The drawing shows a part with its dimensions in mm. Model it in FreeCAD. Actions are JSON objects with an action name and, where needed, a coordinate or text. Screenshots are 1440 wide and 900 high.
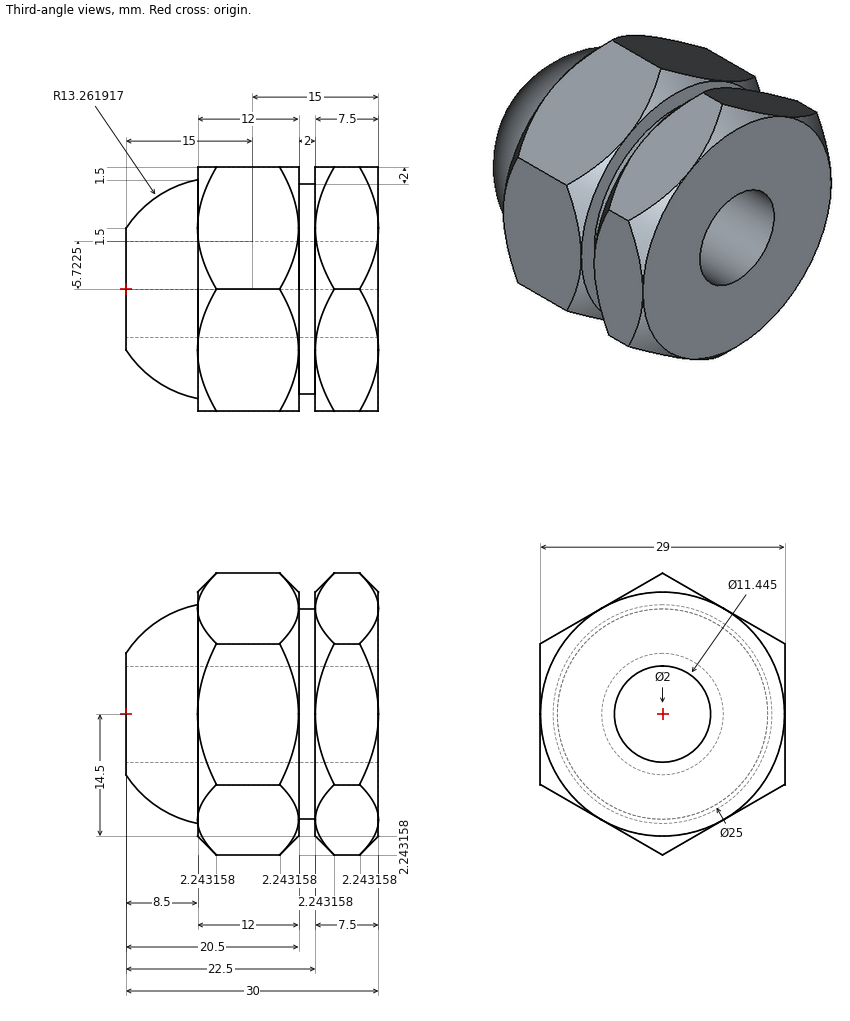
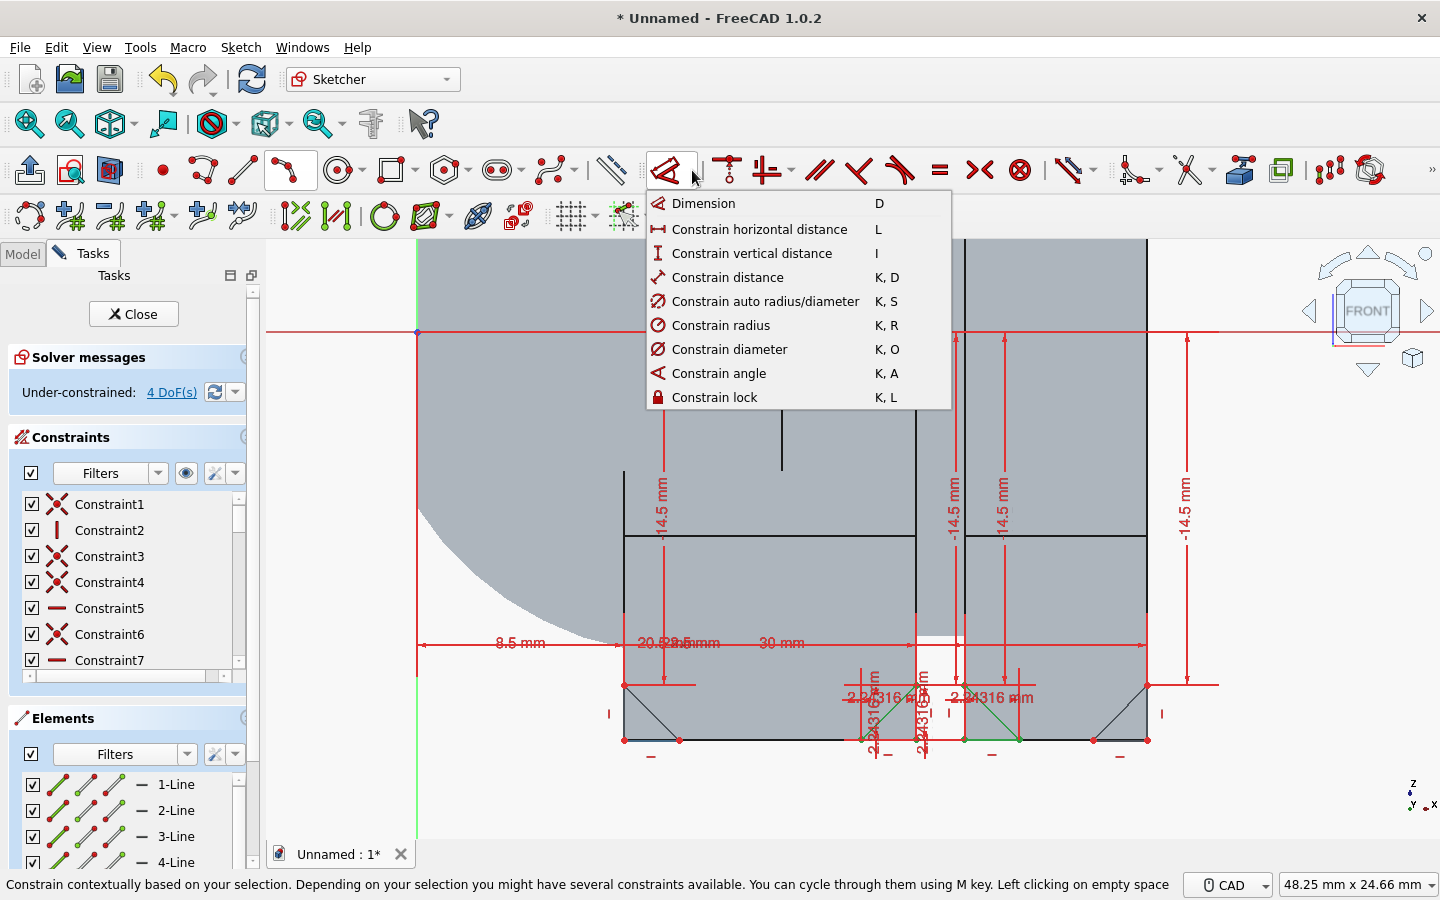
{"action": "left_click", "coordinate": [799, 229]}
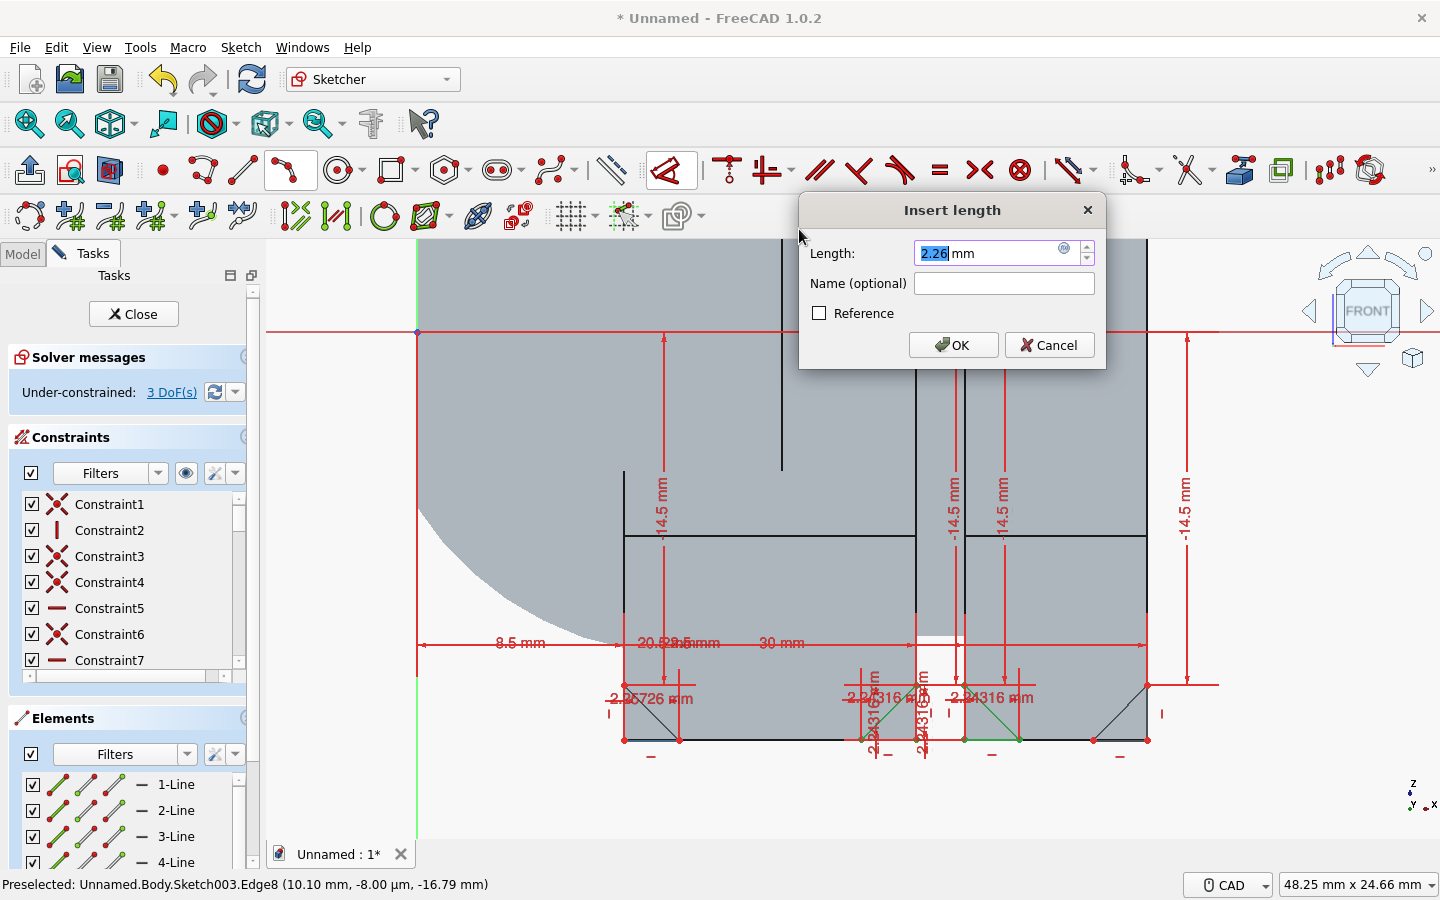
{"action": "type", "text": "2.243158"}
{"action": "key", "text": "Return"}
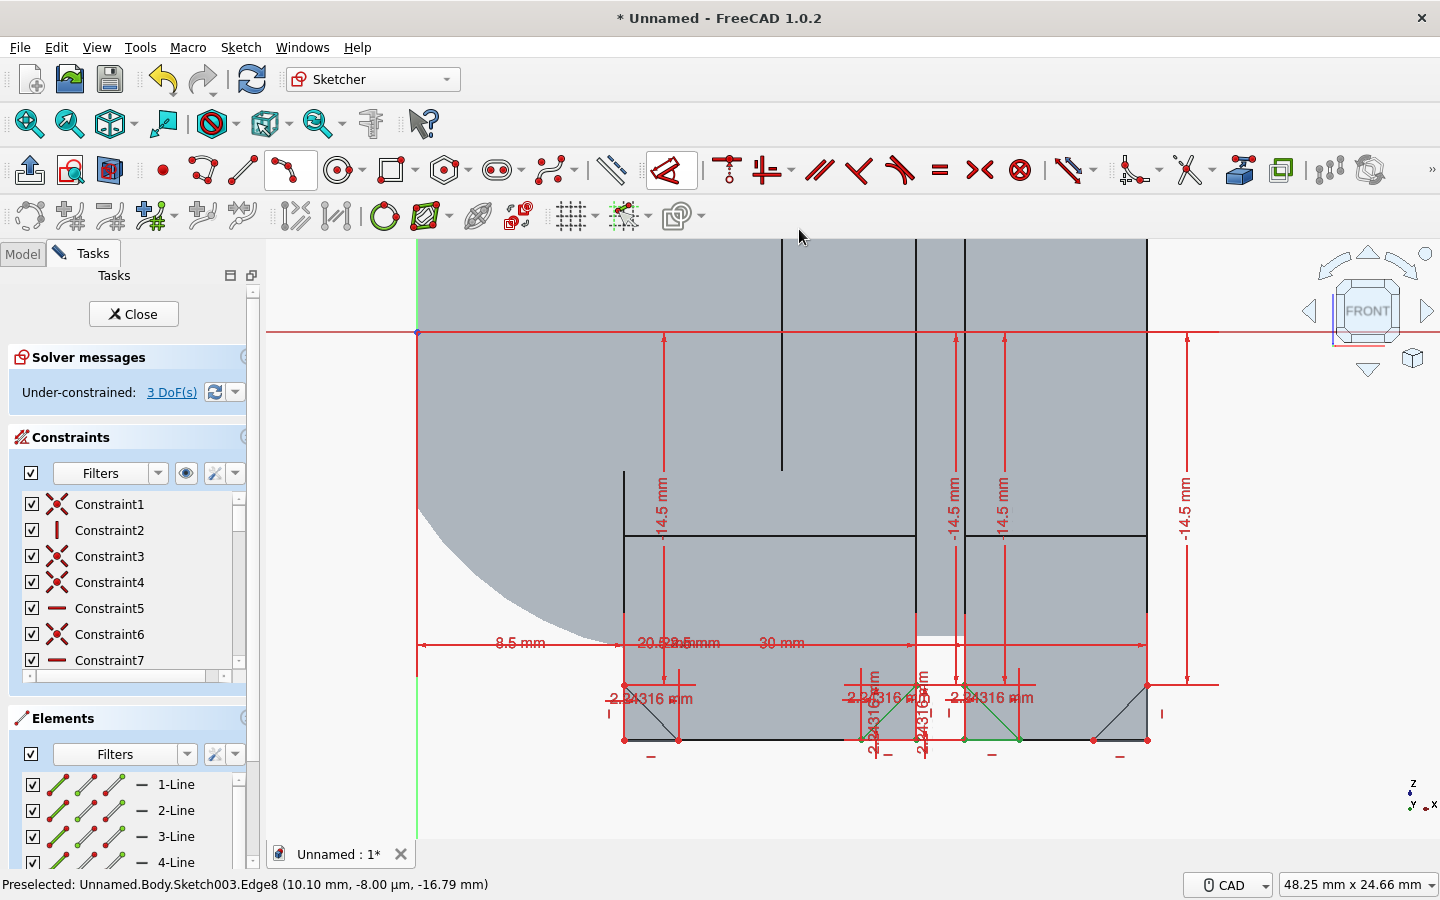
{"action": "left_click", "coordinate": [624, 724]}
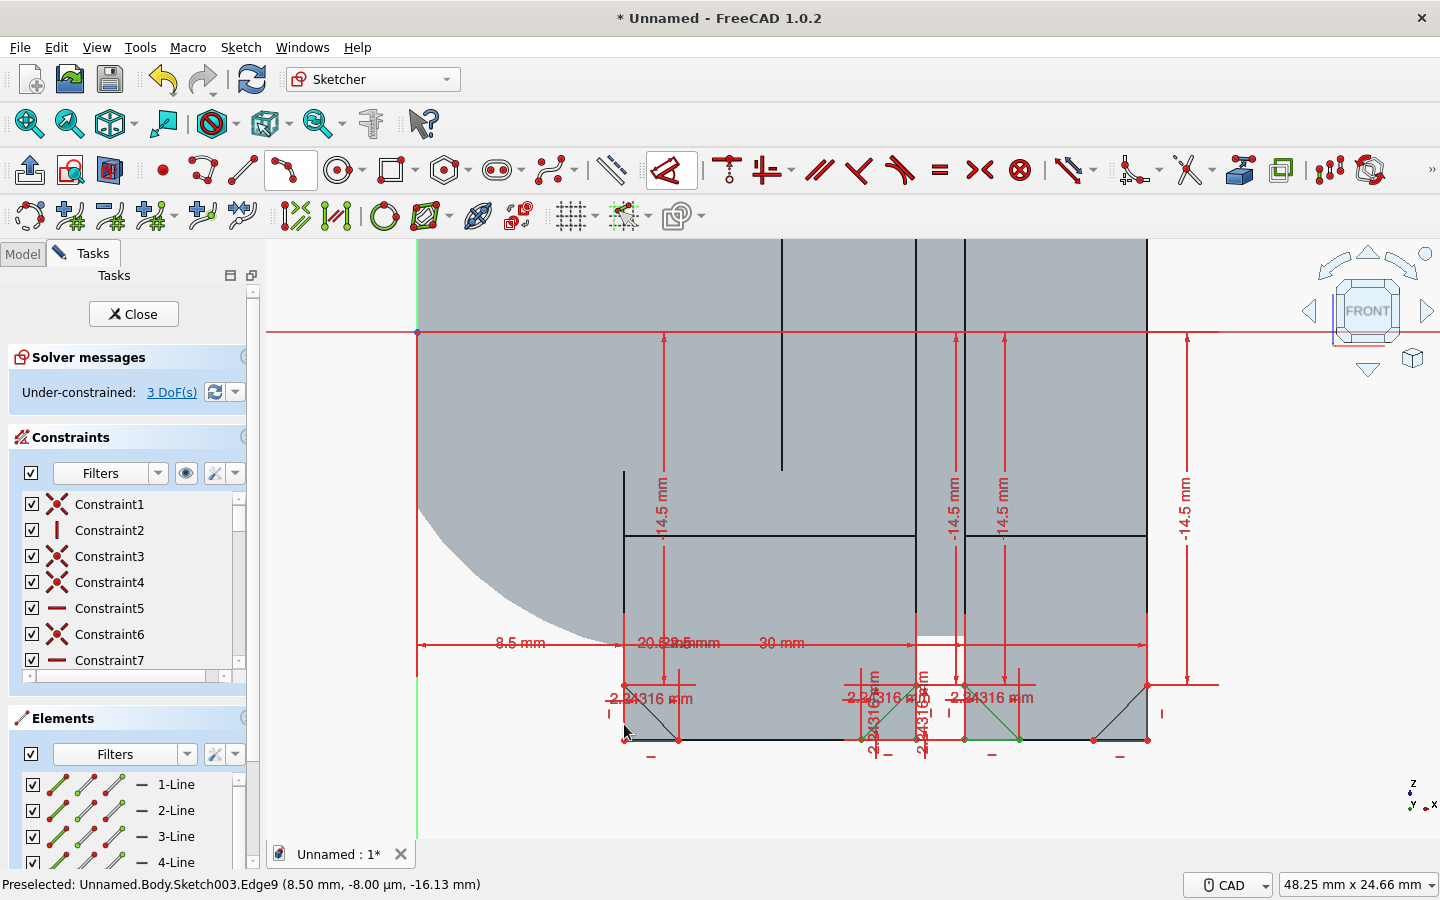
{"action": "left_click", "coordinate": [692, 170]}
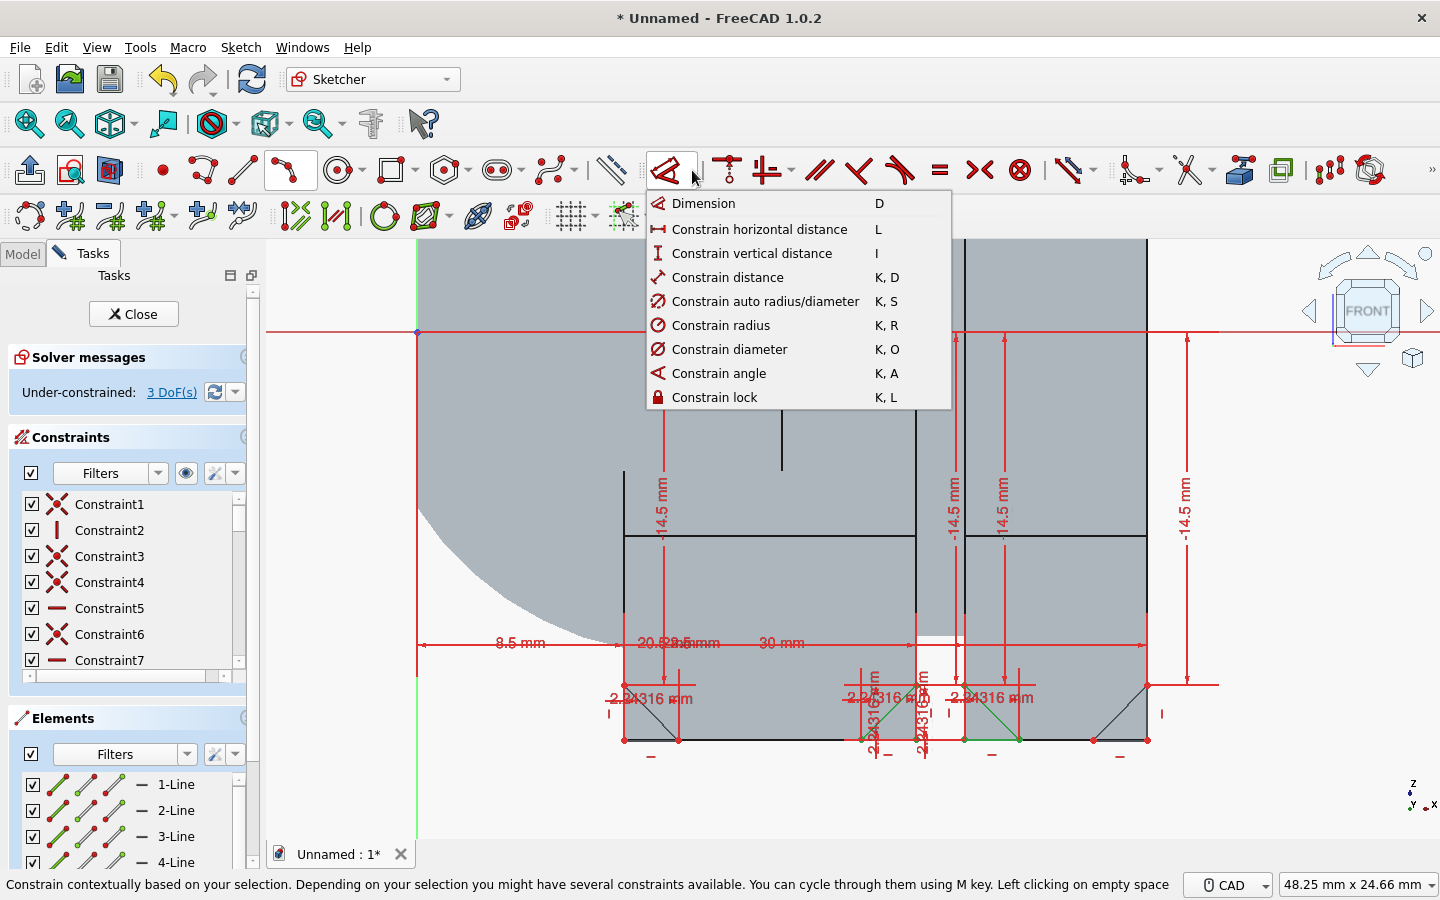
{"action": "left_click", "coordinate": [799, 253]}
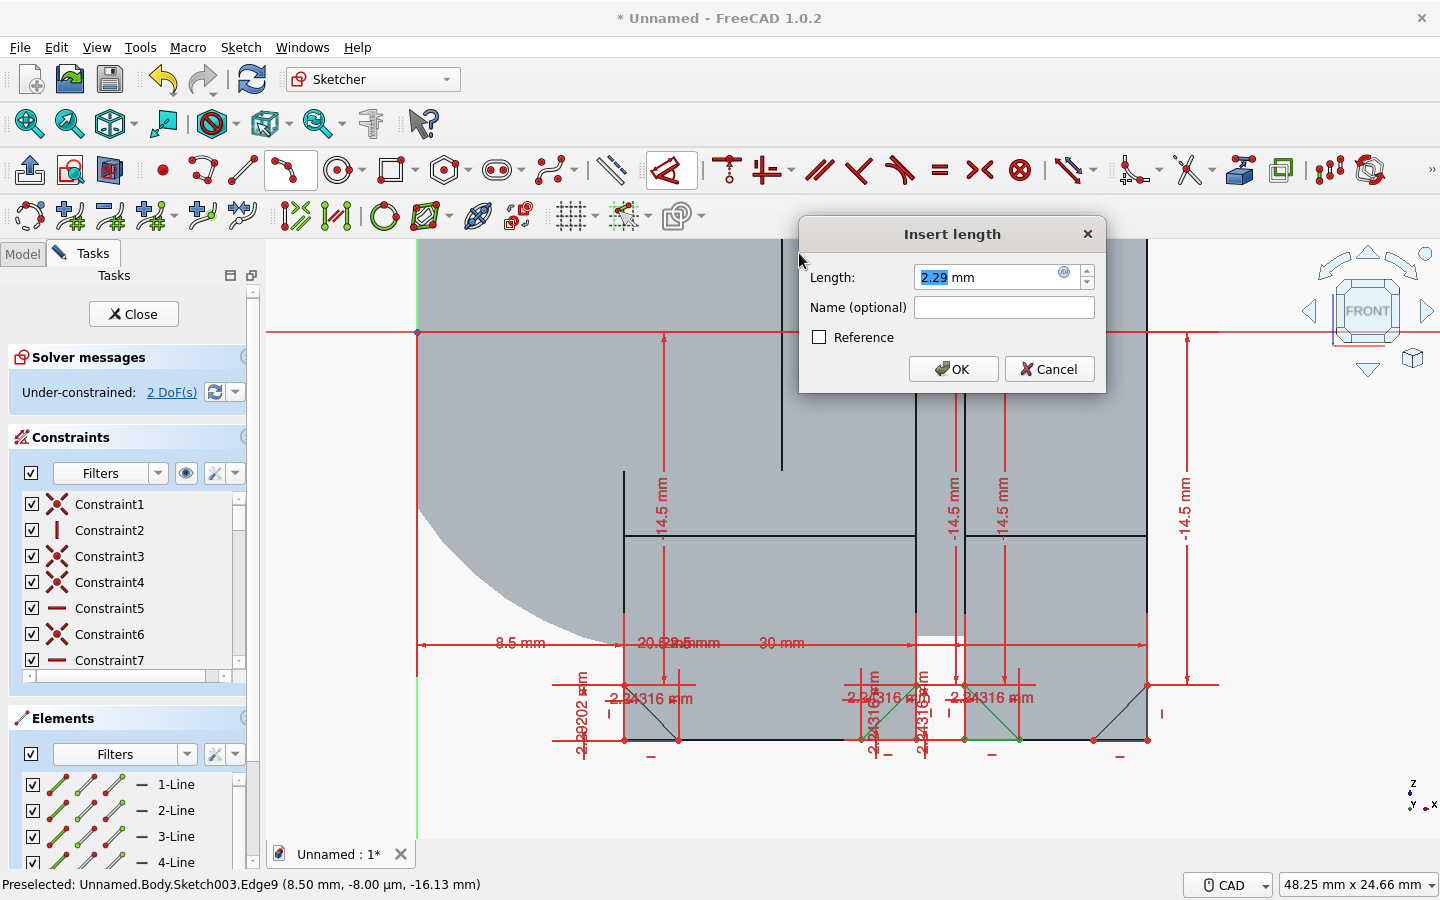
{"action": "type", "text": "2.243158"}
{"action": "key", "text": "Return"}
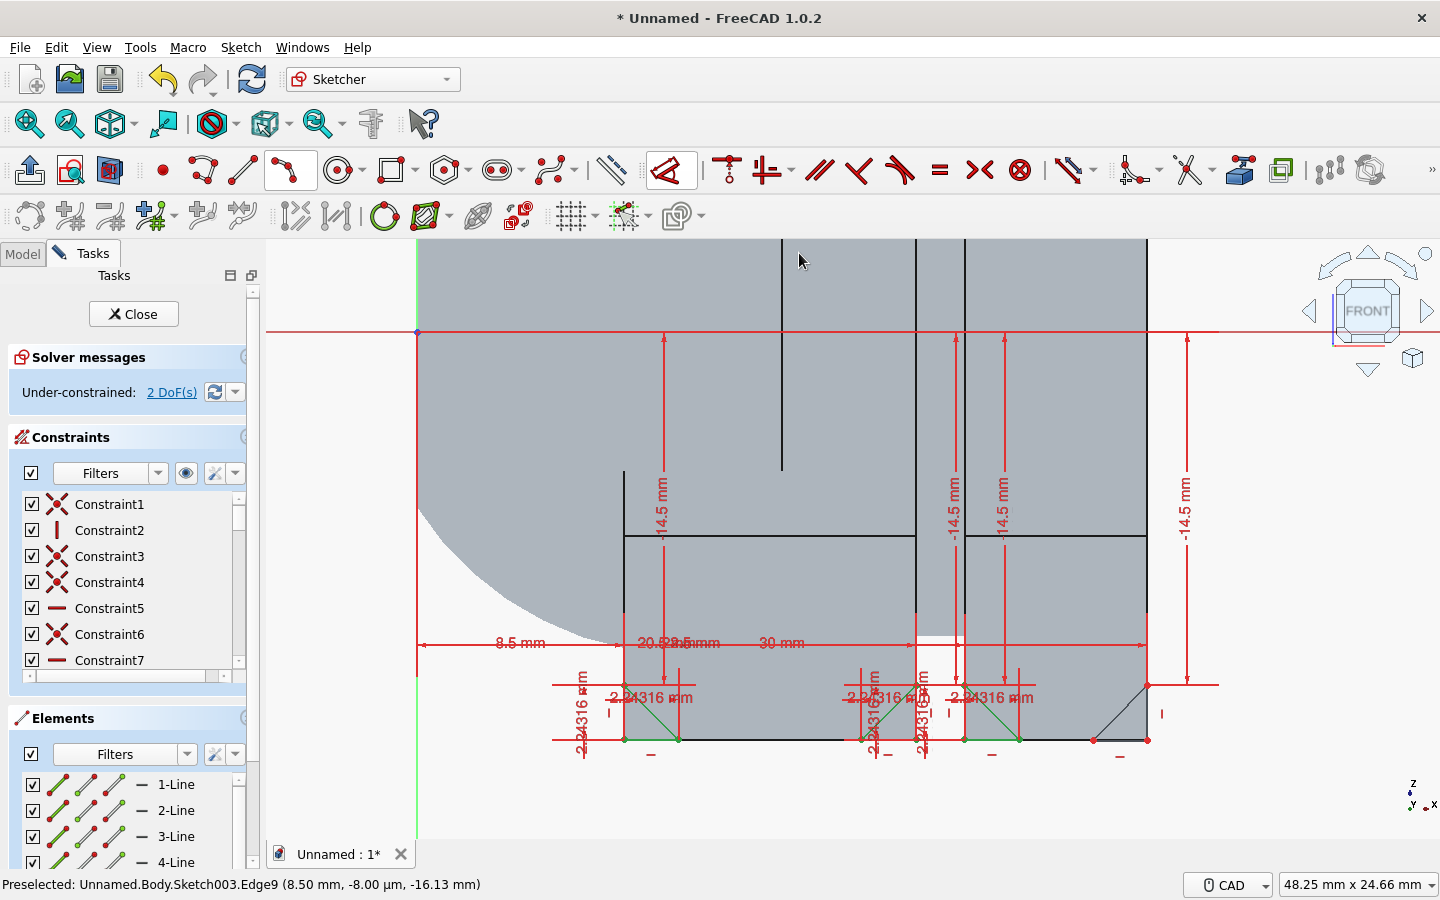
{"action": "left_click", "coordinate": [1147, 702]}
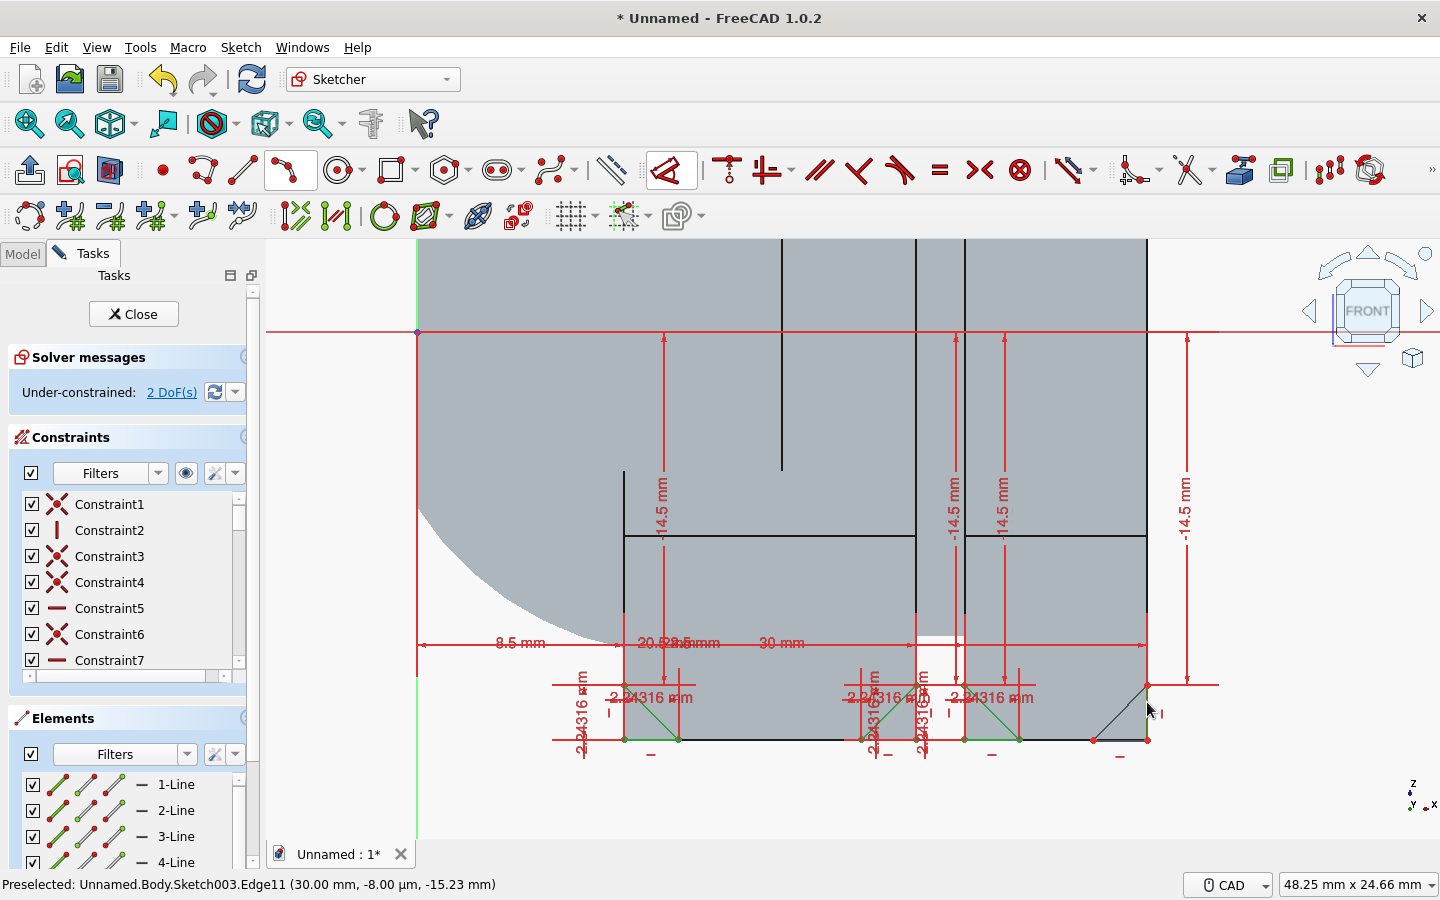
{"action": "key", "text": "i"}